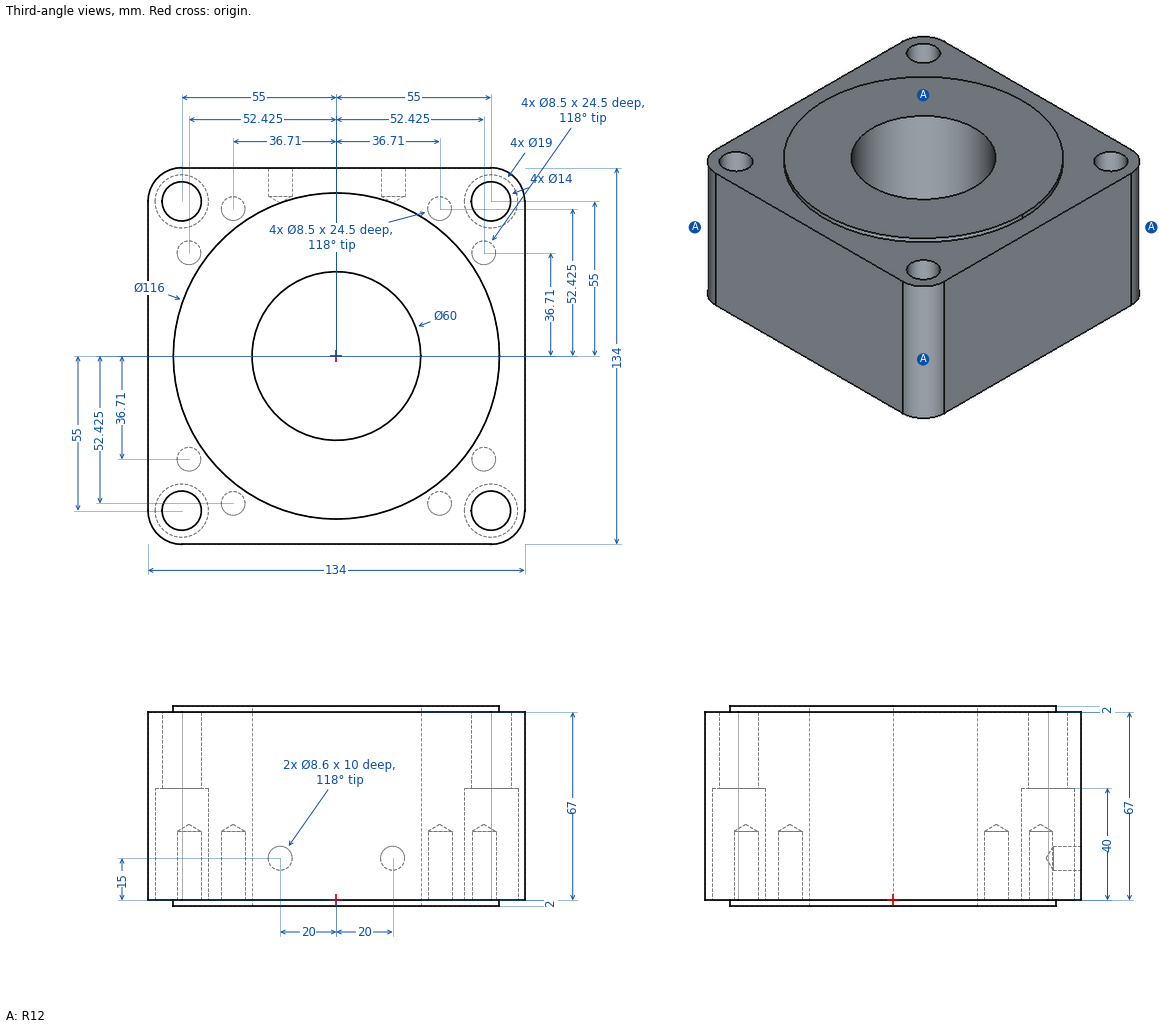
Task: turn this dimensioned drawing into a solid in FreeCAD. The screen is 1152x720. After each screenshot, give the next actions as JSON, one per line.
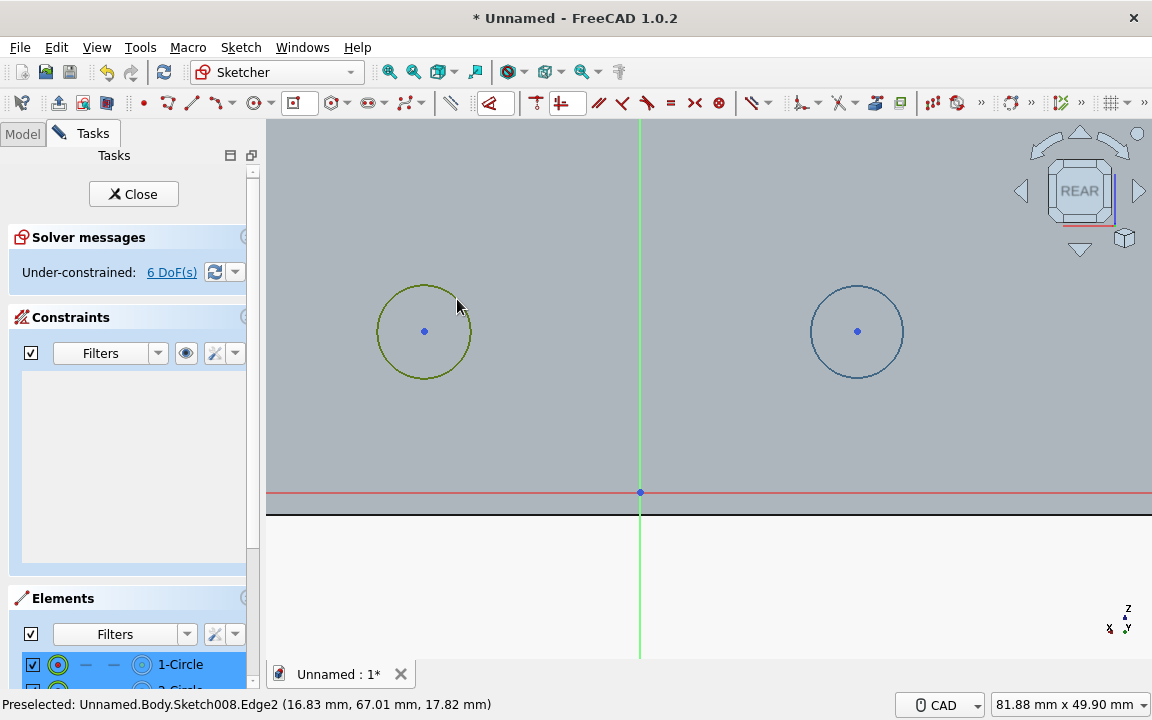
{"action": "left_click", "coordinate": [672, 104]}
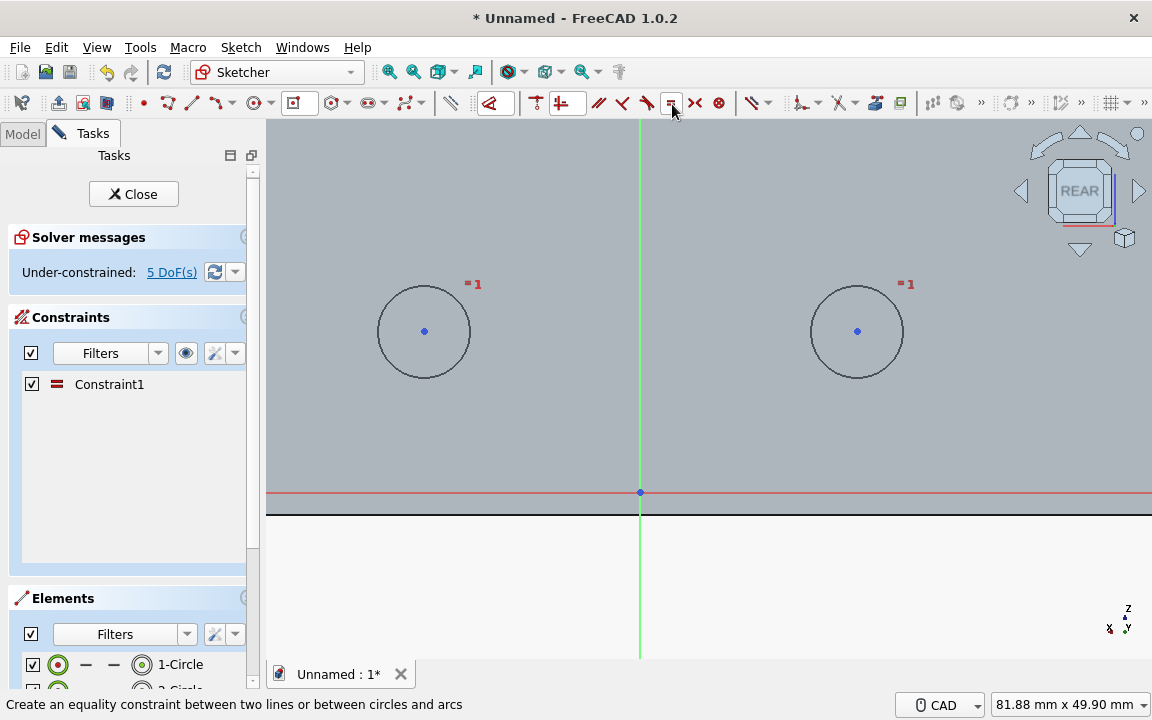
{"action": "left_click", "coordinate": [857, 332]}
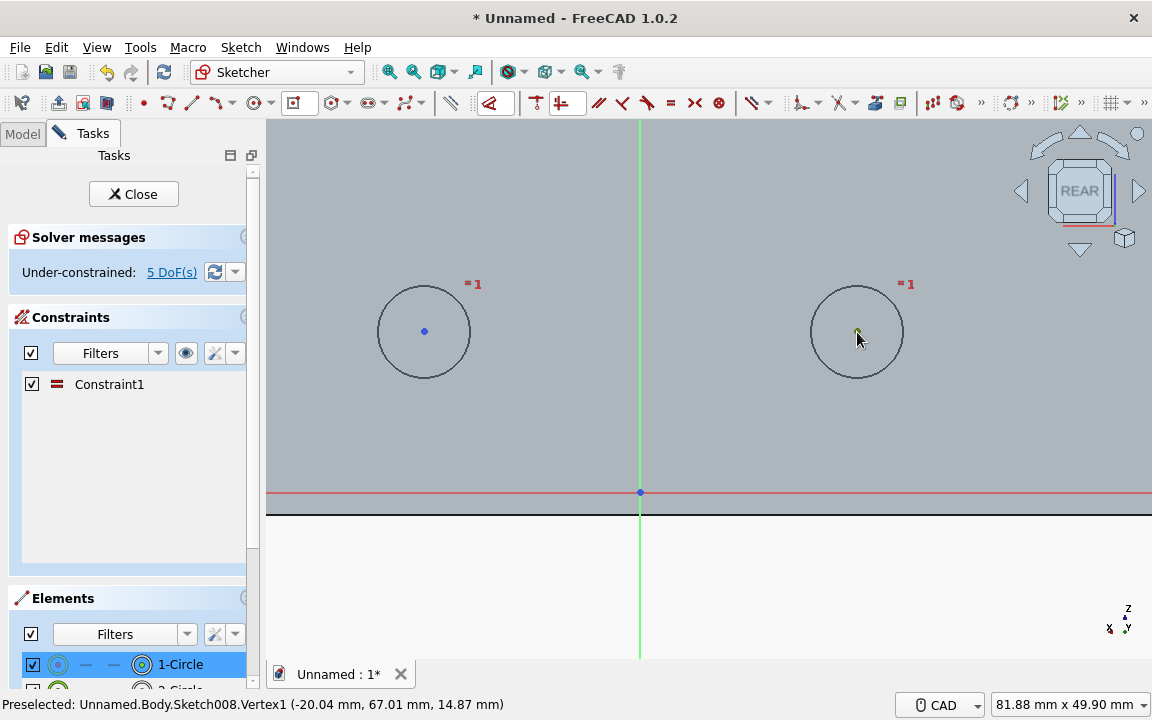
{"action": "left_click", "coordinate": [424, 332]}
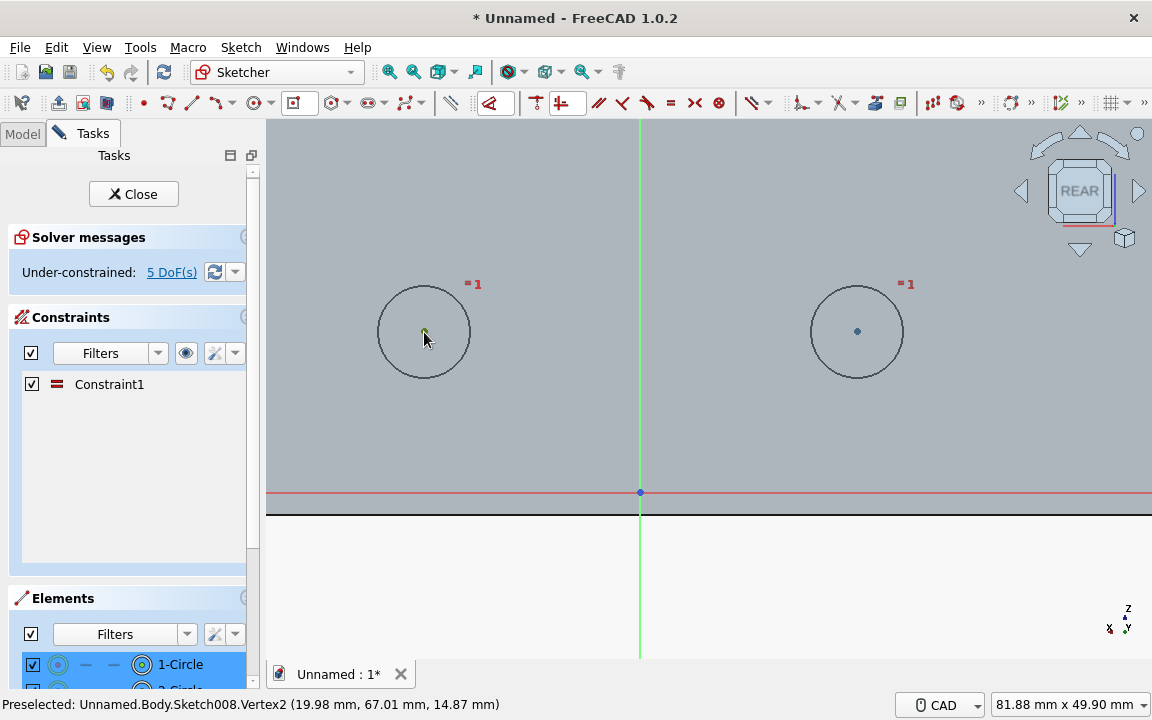
{"action": "left_click", "coordinate": [580, 104]}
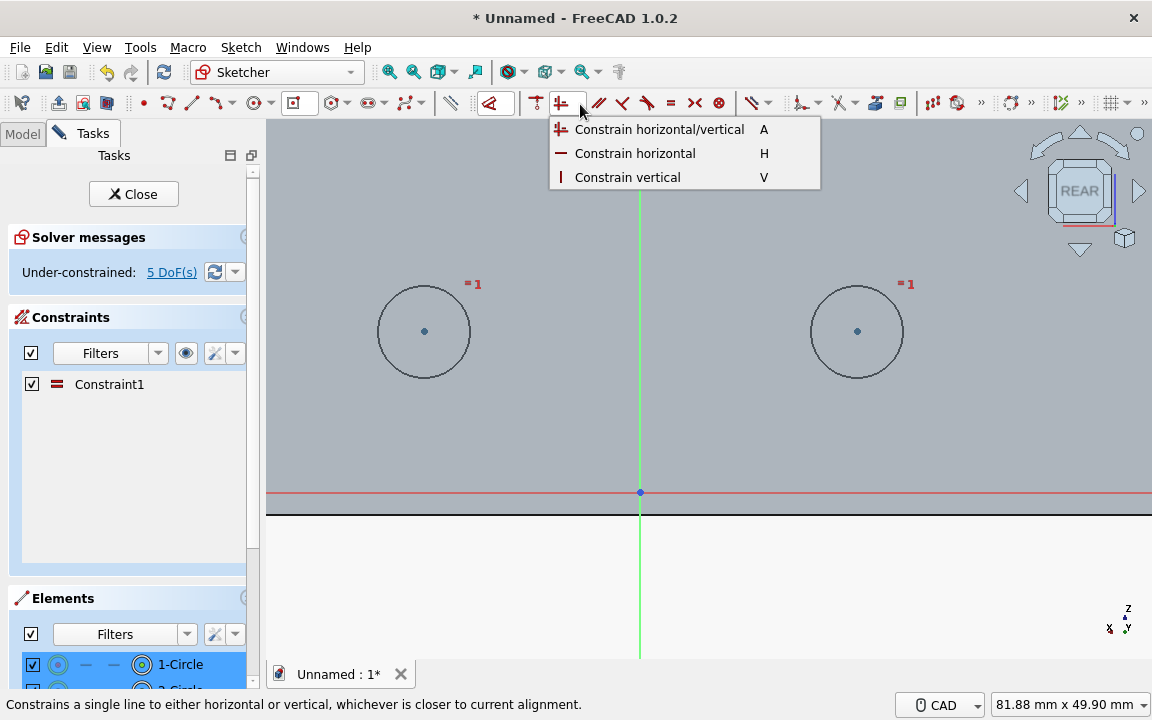
{"action": "left_click", "coordinate": [685, 153]}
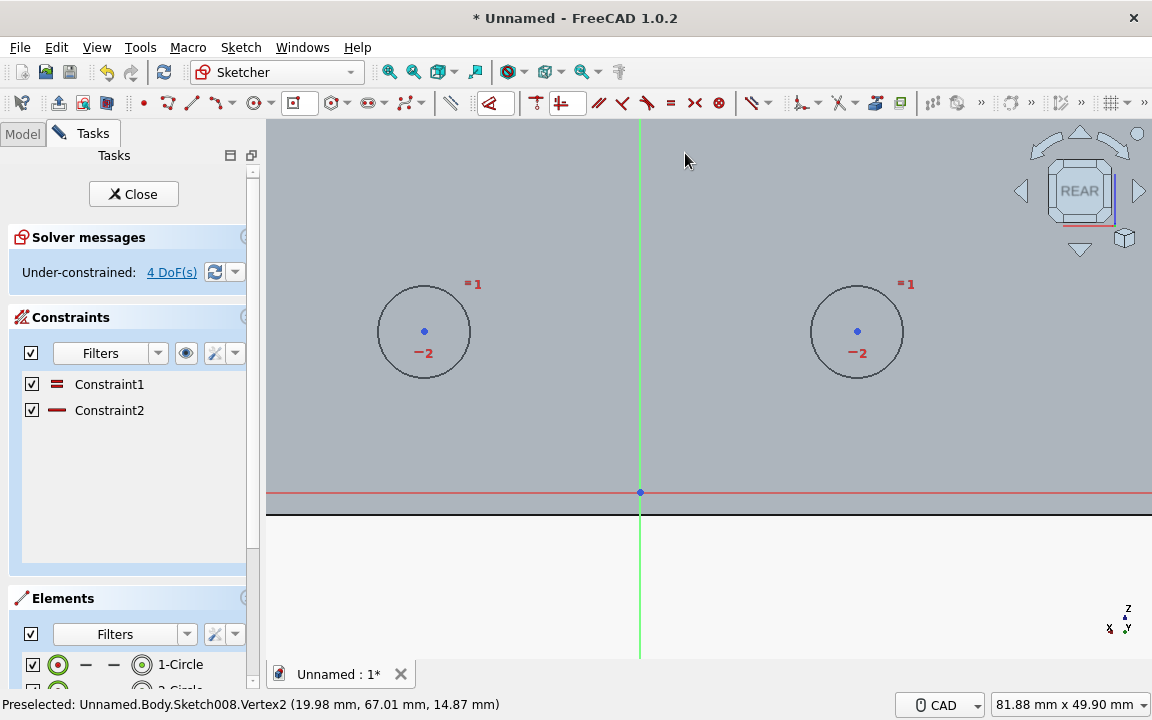
{"action": "left_click", "coordinate": [889, 299]}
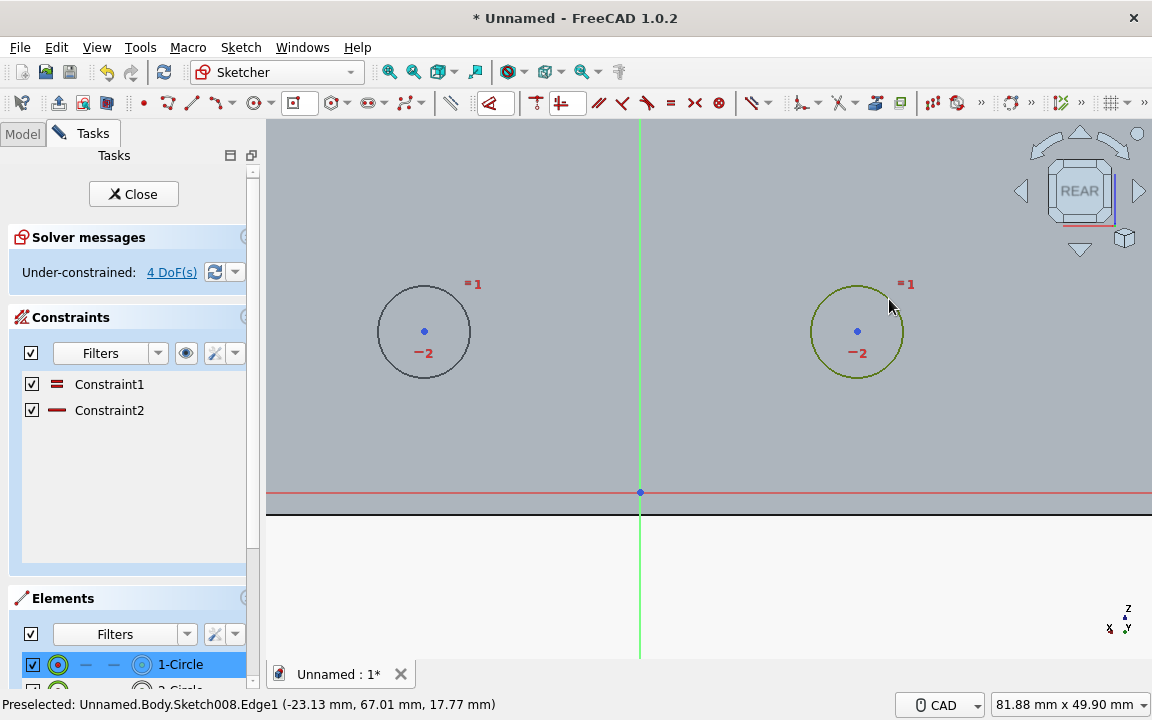
{"action": "left_click", "coordinate": [508, 104]}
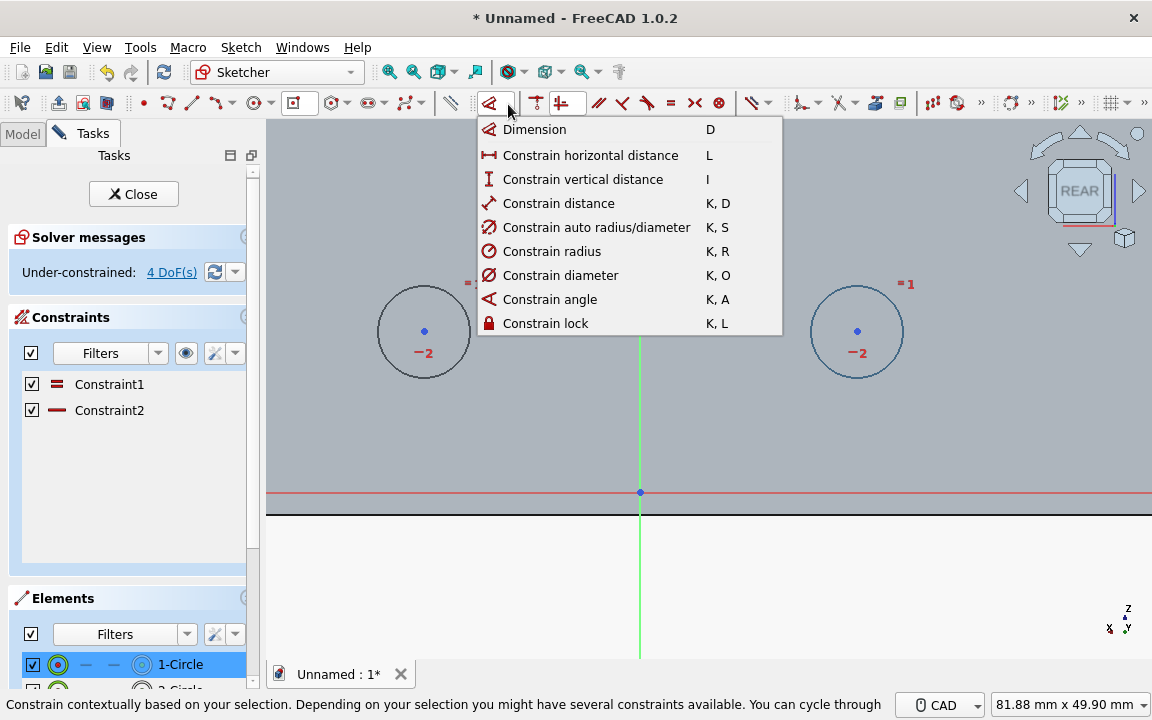
{"action": "left_click", "coordinate": [630, 275]}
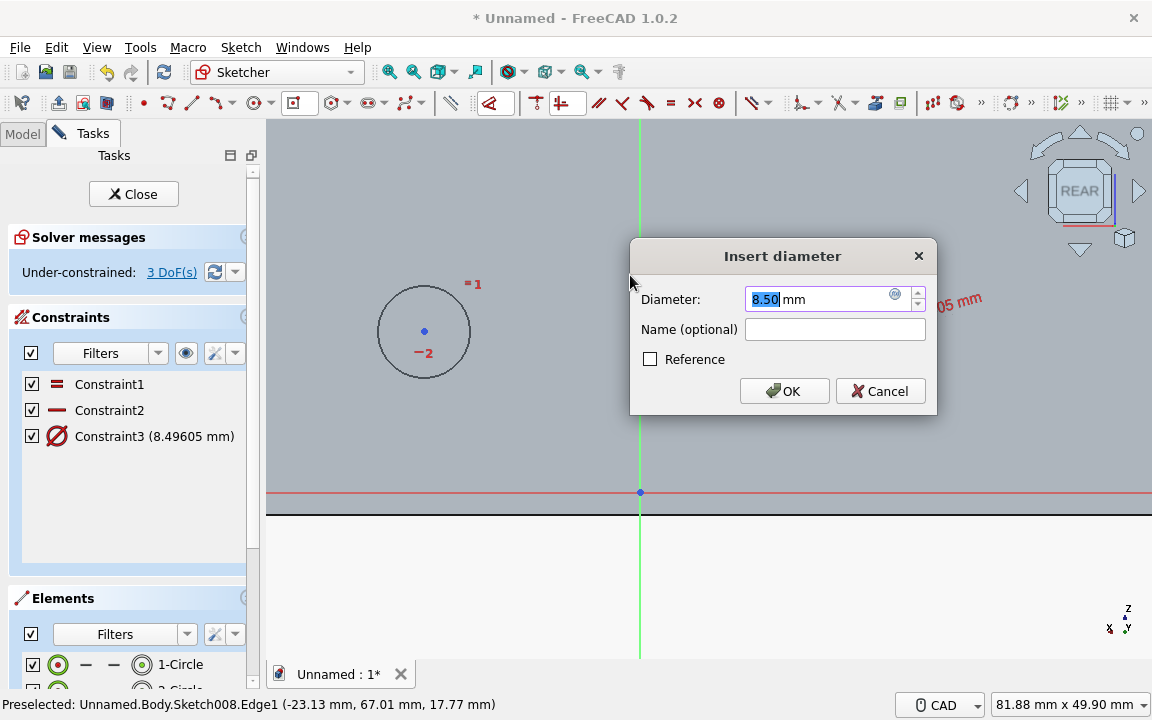
{"action": "type", "text": "8.6"}
{"action": "key", "text": "Return"}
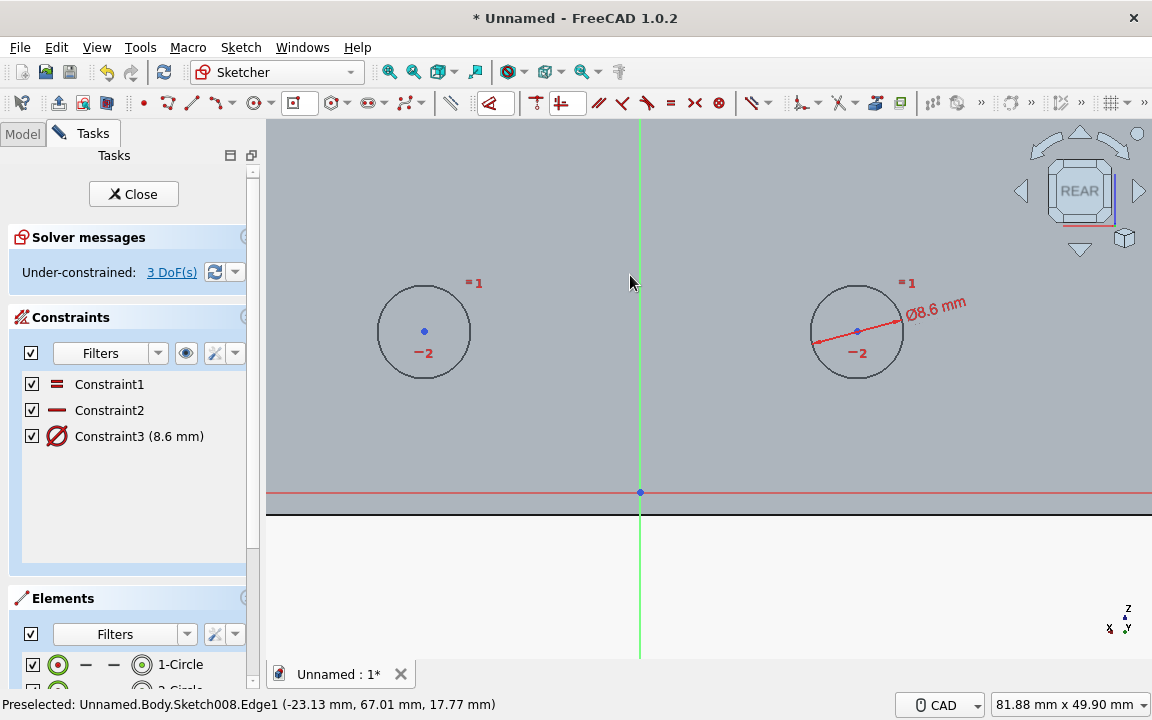
{"action": "left_click", "coordinate": [857, 332]}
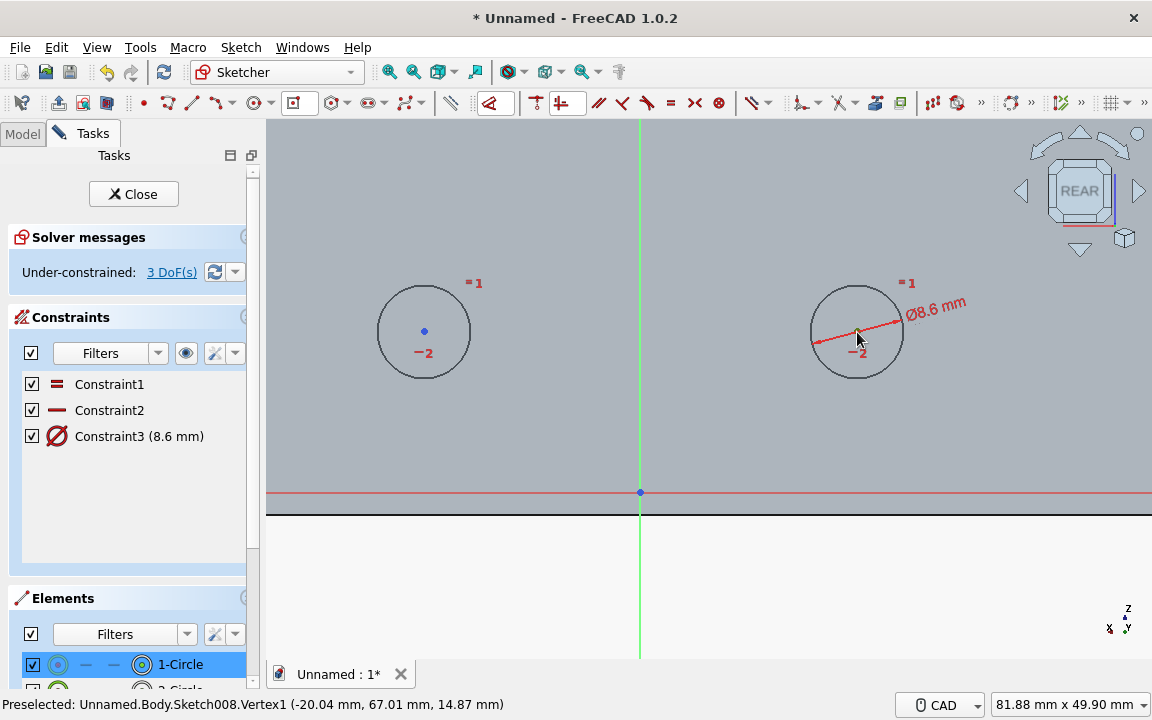
{"action": "key", "text": "l"}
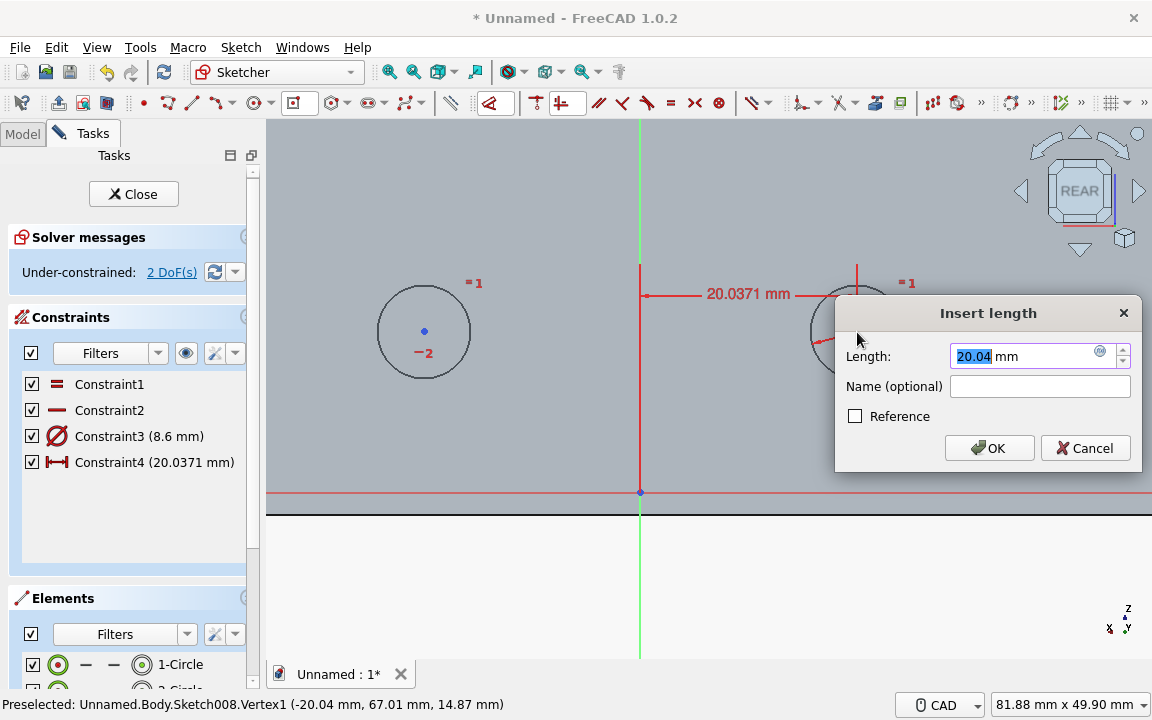
{"action": "type", "text": "20"}
{"action": "key", "text": "Return"}